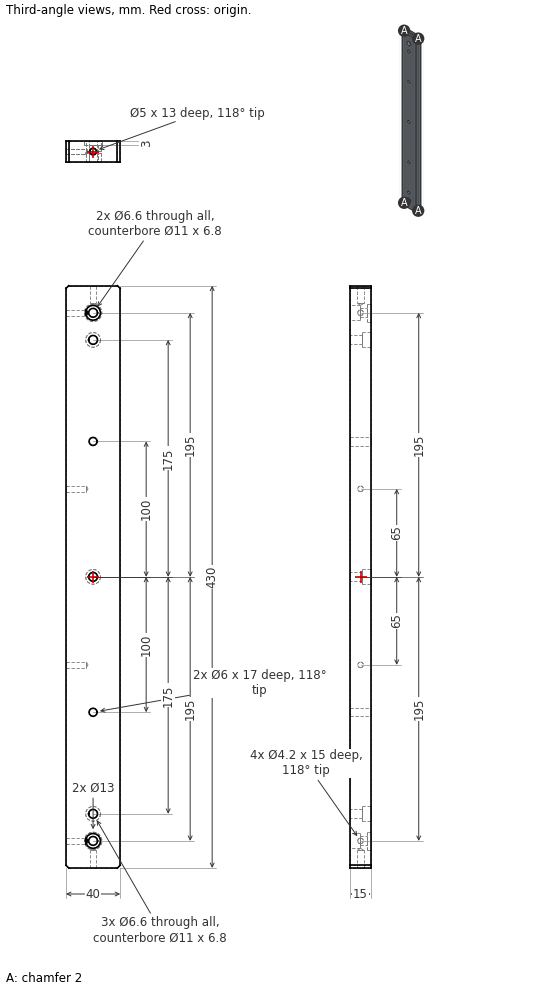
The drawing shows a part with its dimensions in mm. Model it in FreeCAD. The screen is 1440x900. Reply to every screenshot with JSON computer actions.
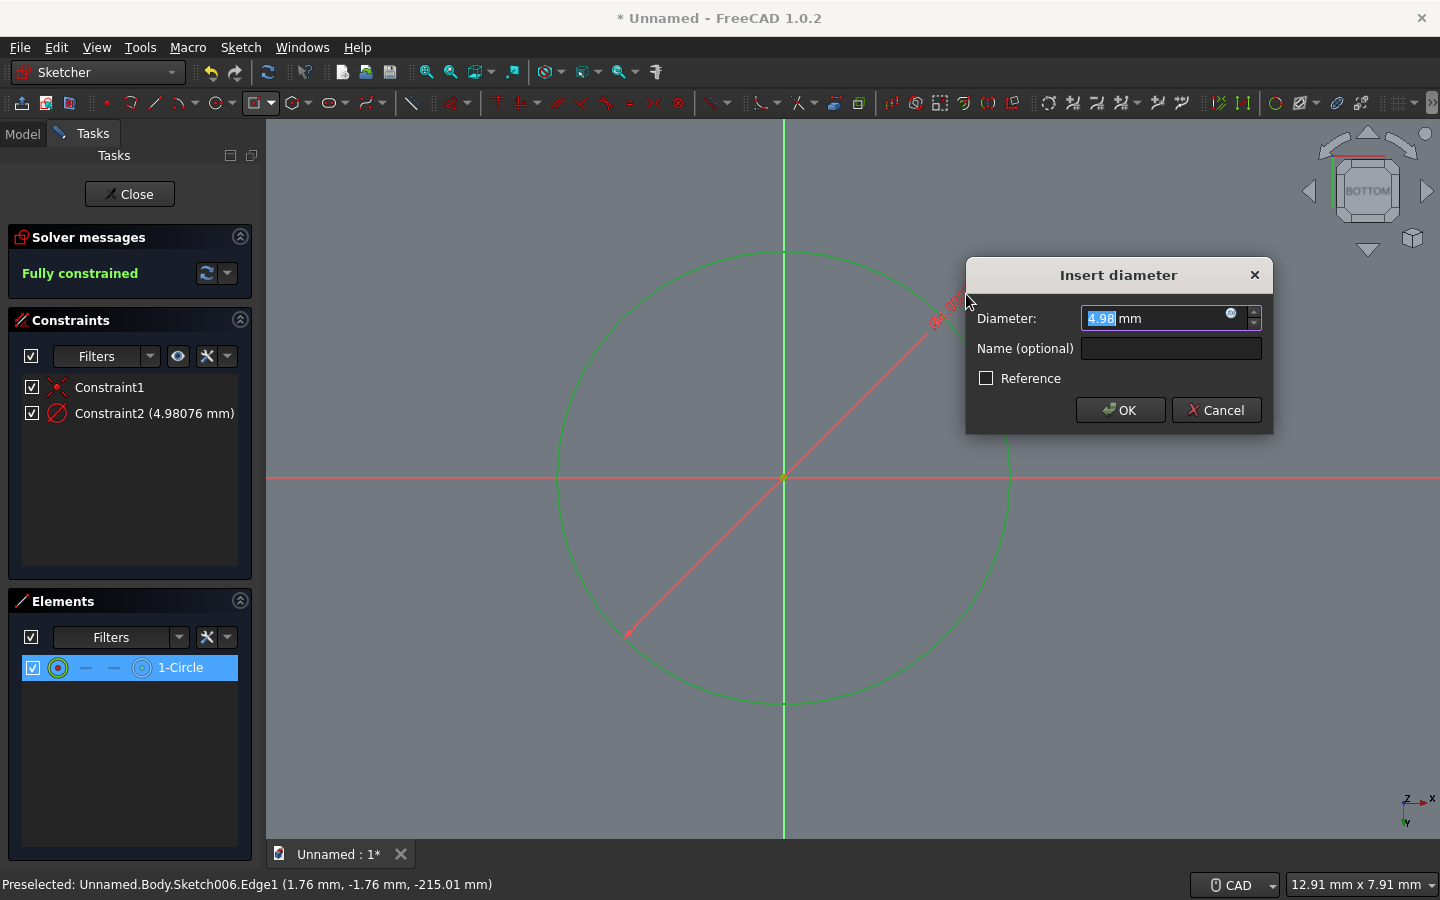
{"action": "type", "text": "5"}
{"action": "key", "text": "Return"}
{"action": "key", "text": "Escape"}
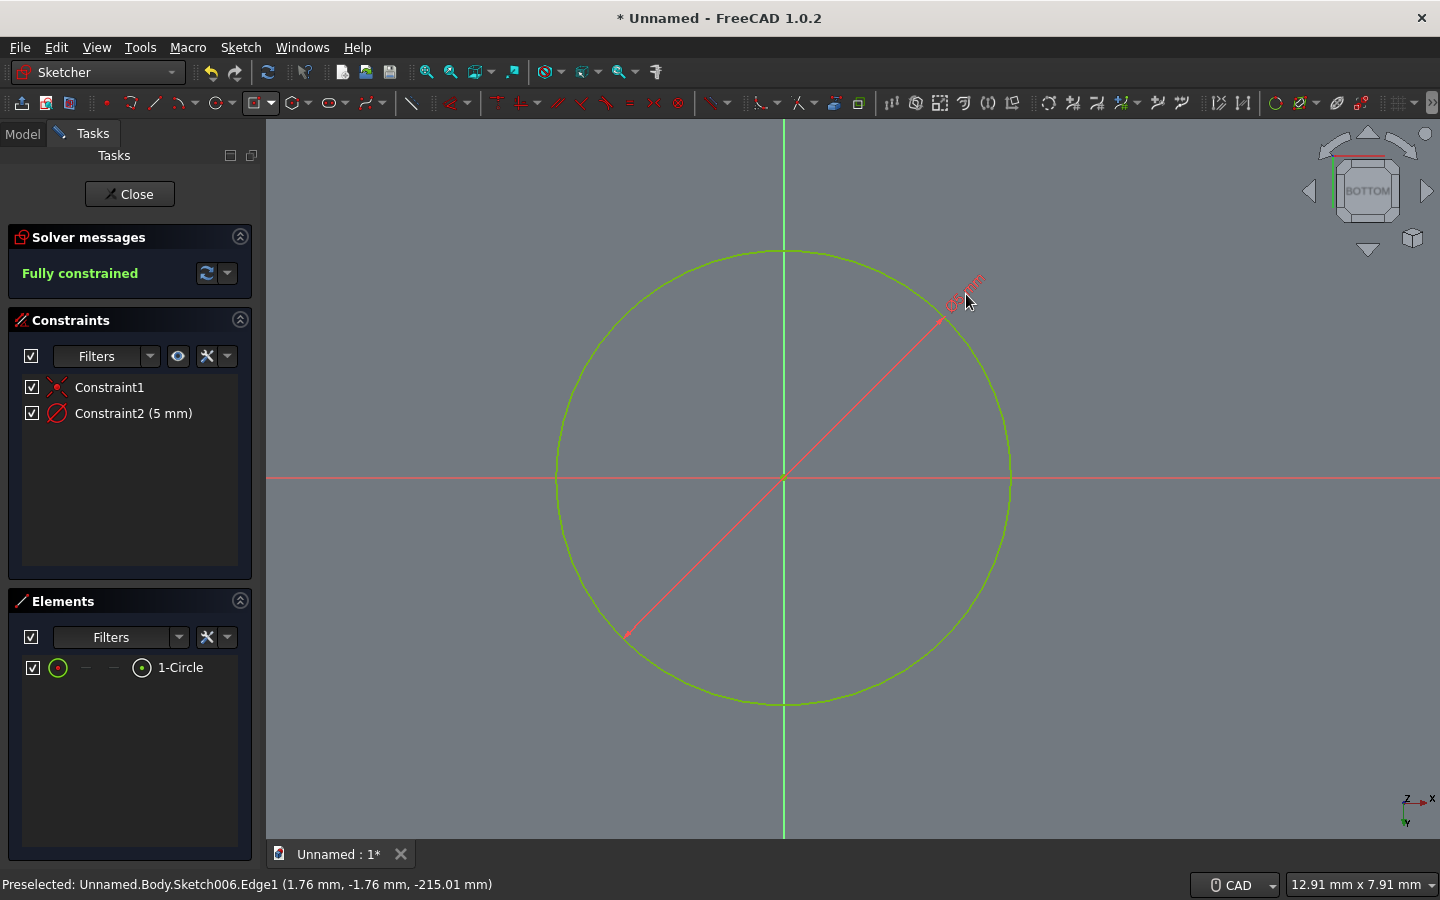
{"action": "left_click", "coordinate": [130, 194]}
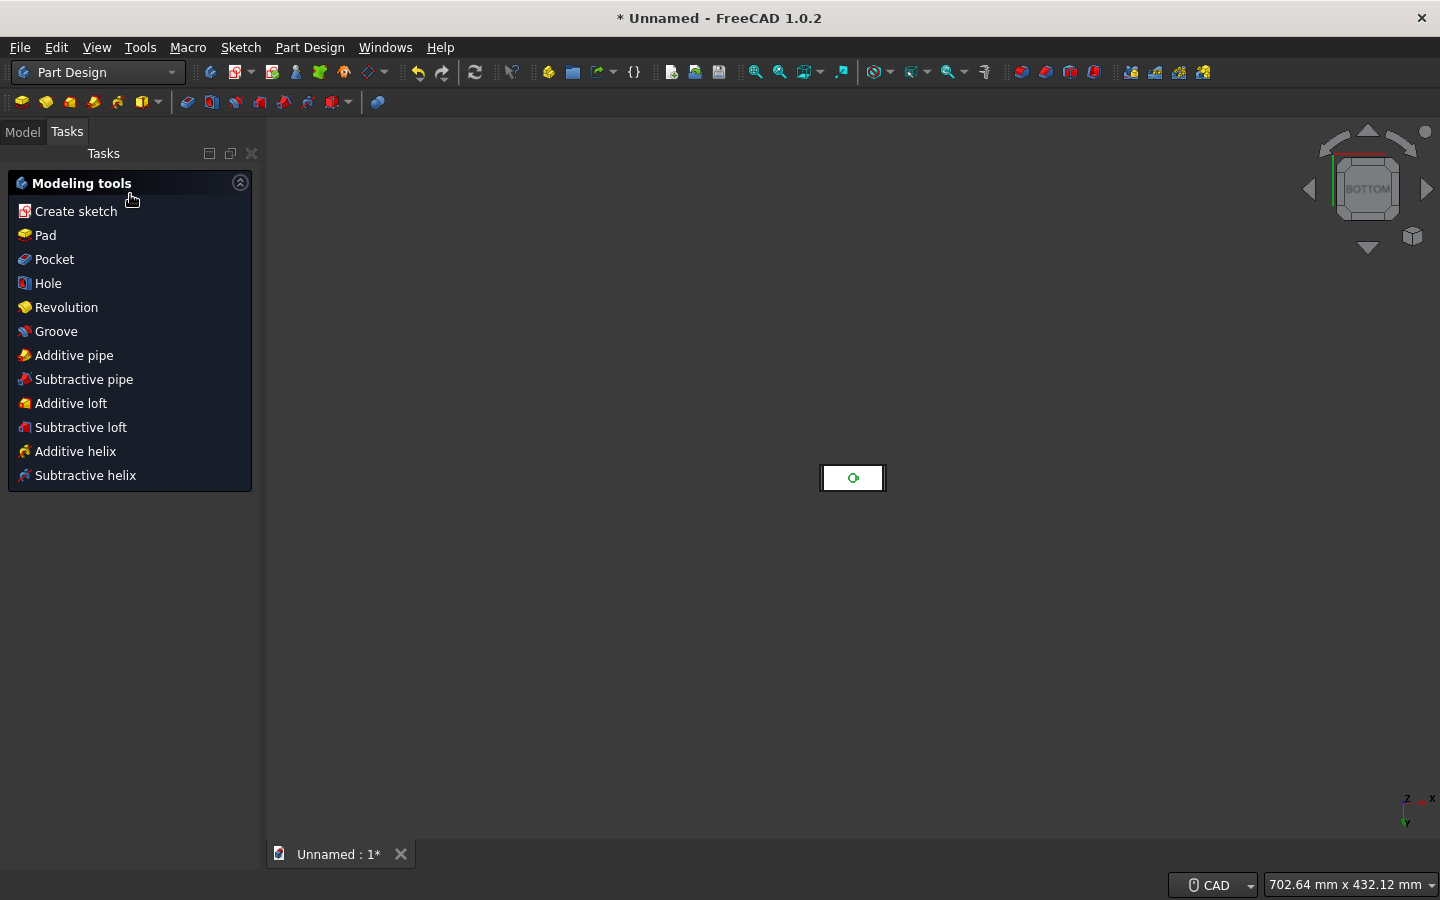
{"action": "left_click", "coordinate": [212, 102]}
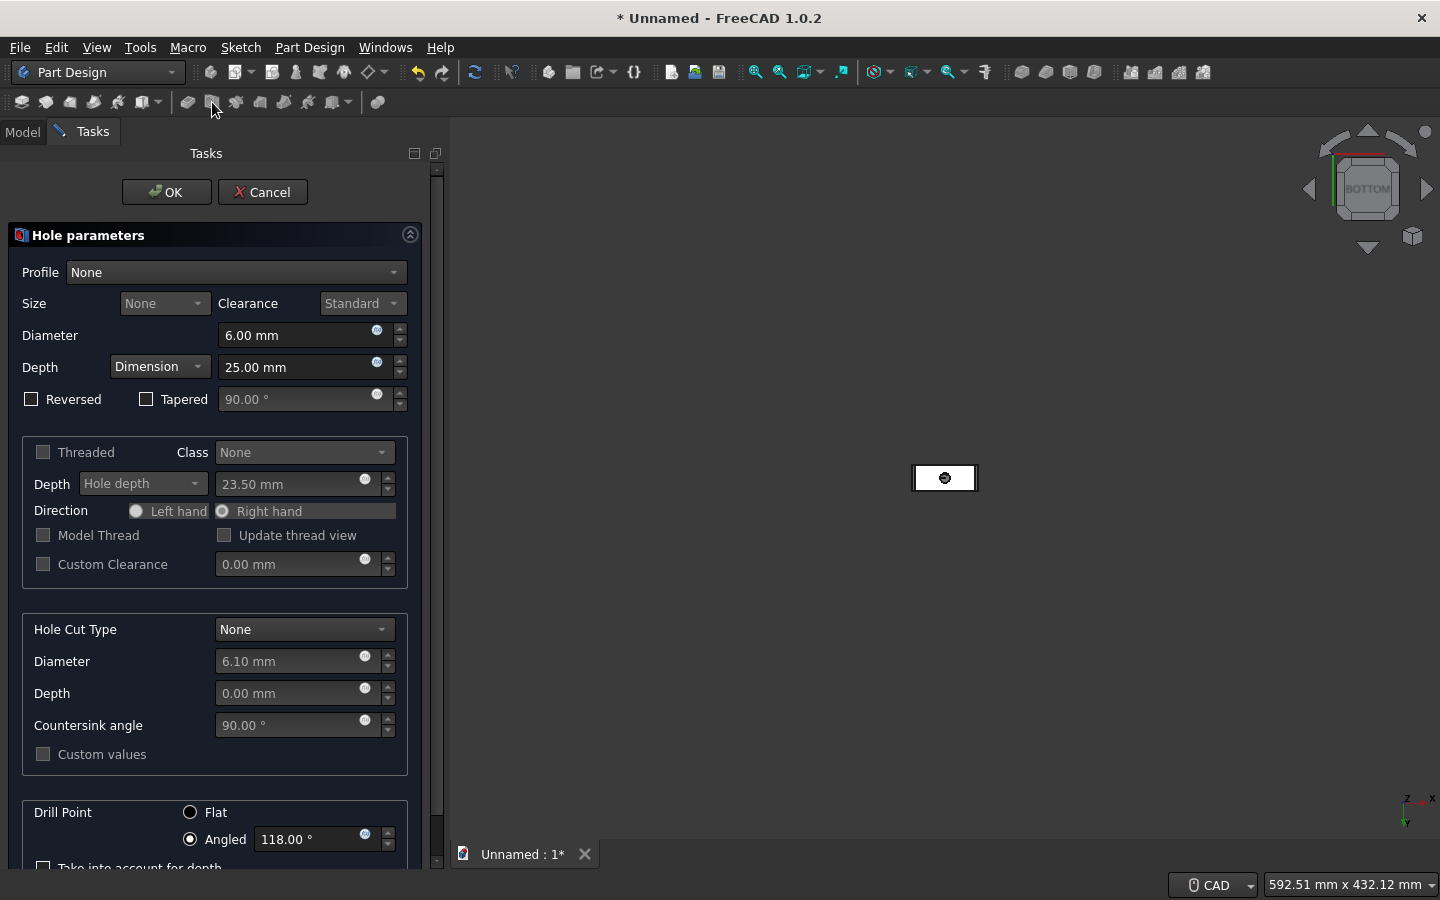
{"action": "triple_click", "coordinate": [305, 335]}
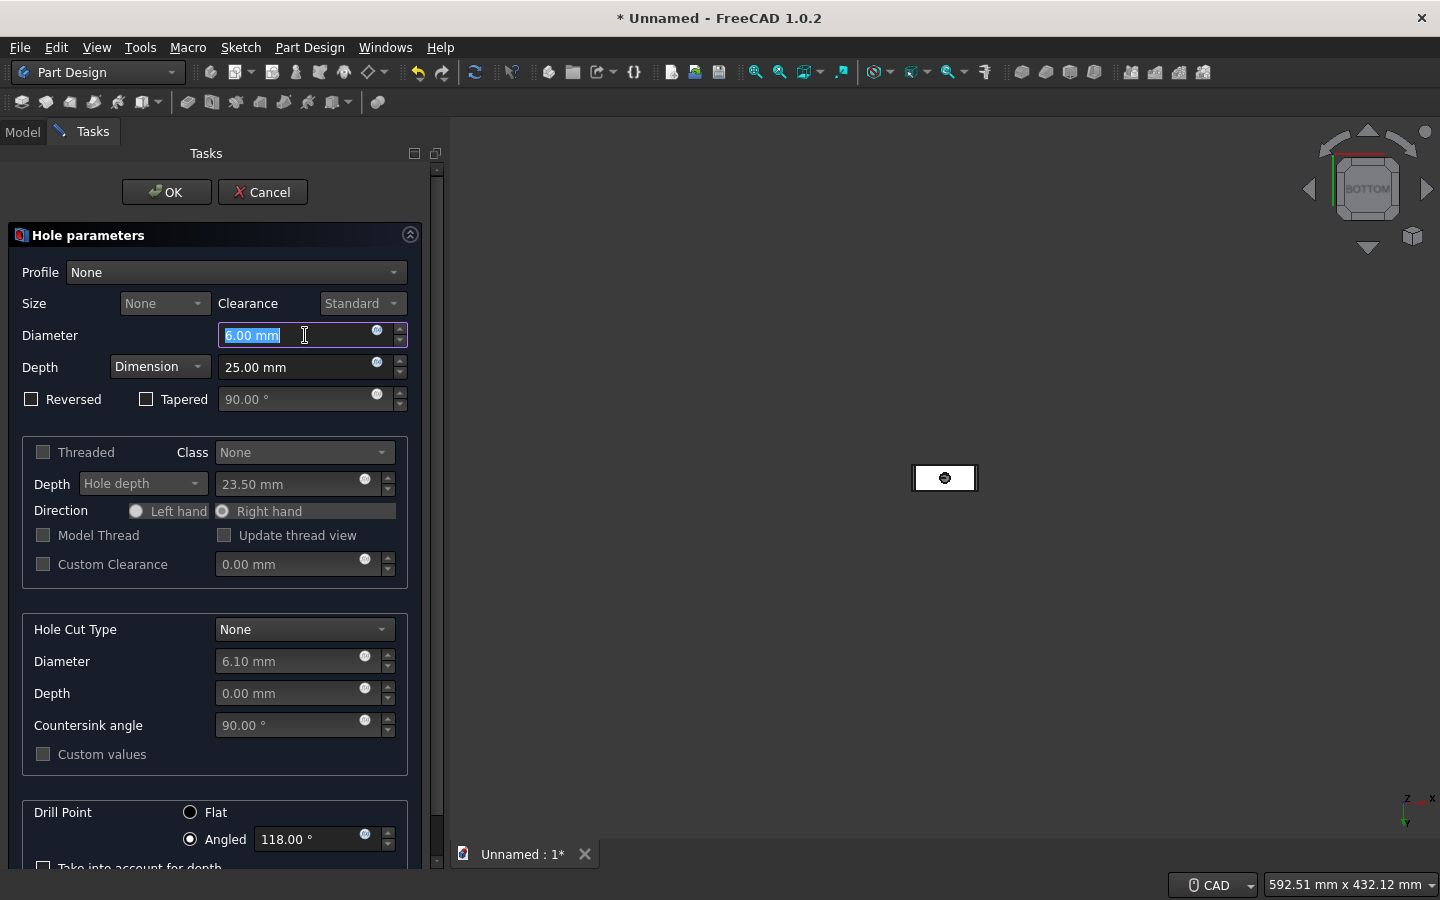
{"action": "type", "text": "5"}
{"action": "key", "text": "Tab"}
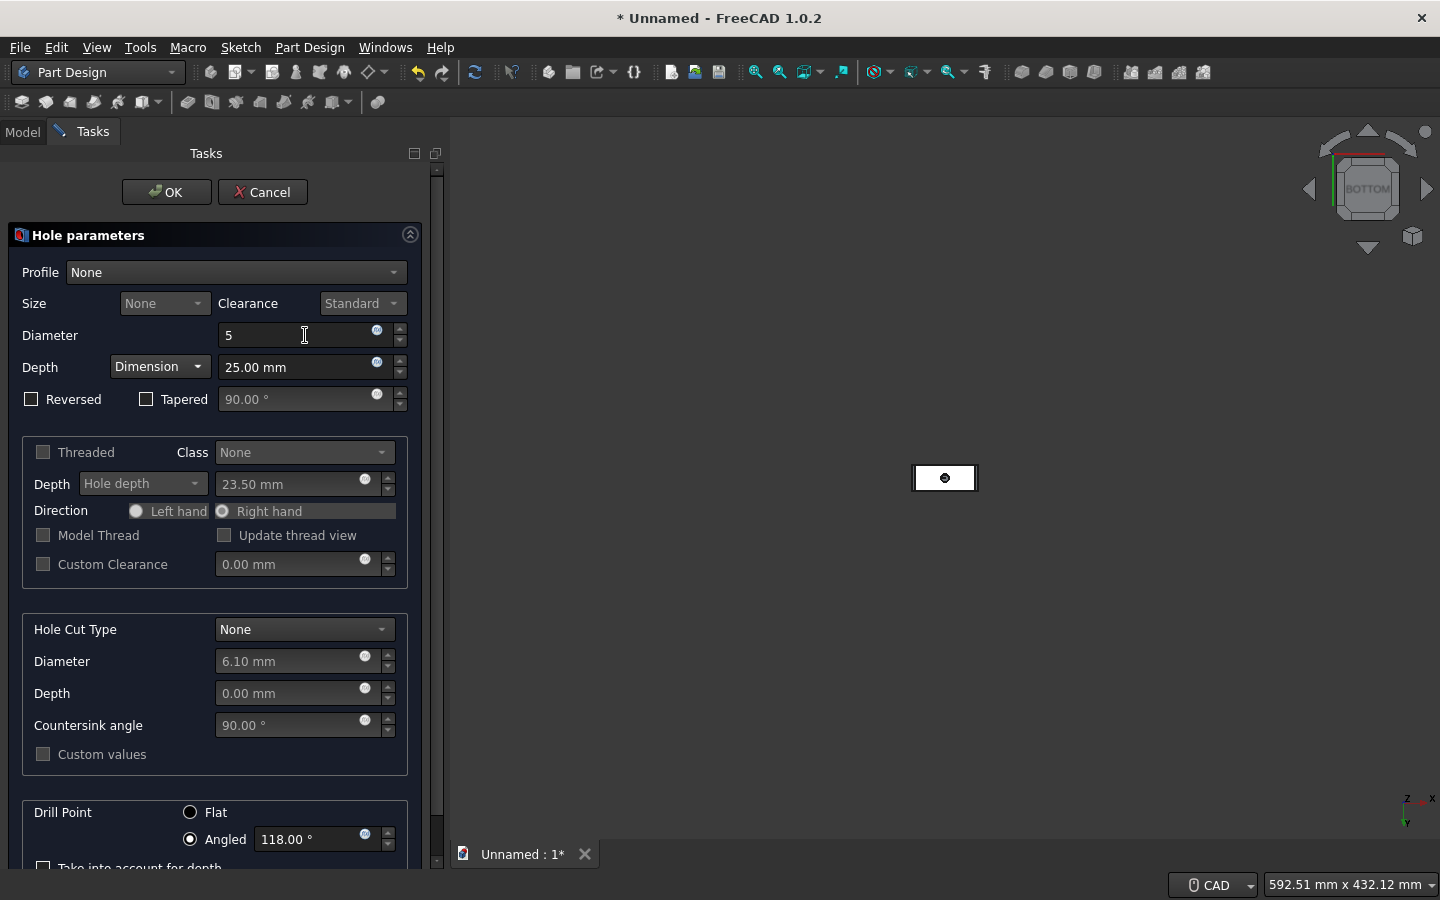
{"action": "triple_click", "coordinate": [305, 367]}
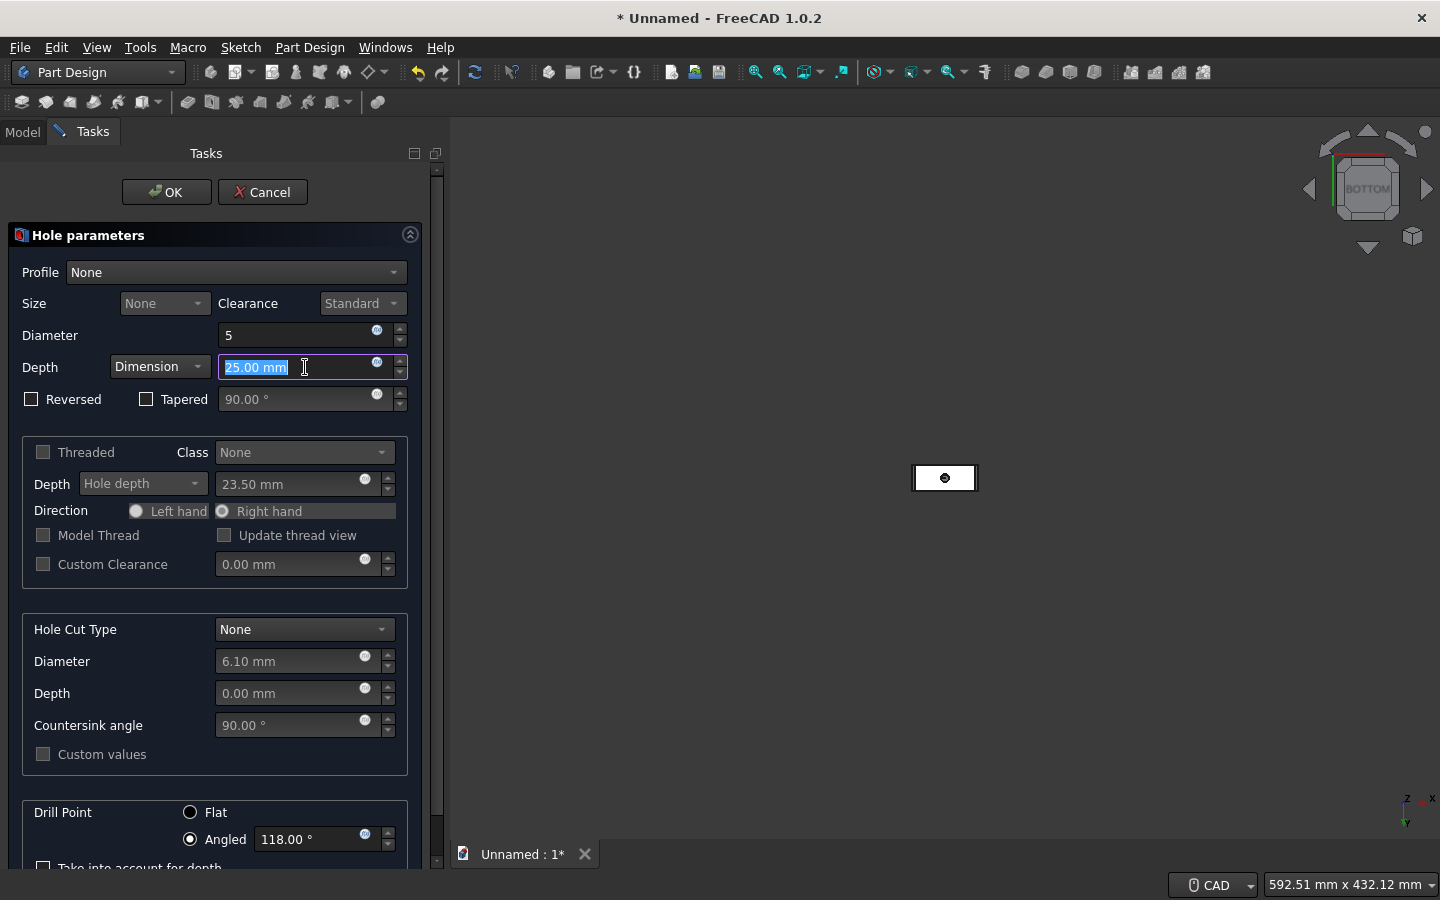
{"action": "type", "text": "13"}
{"action": "key", "text": "Tab"}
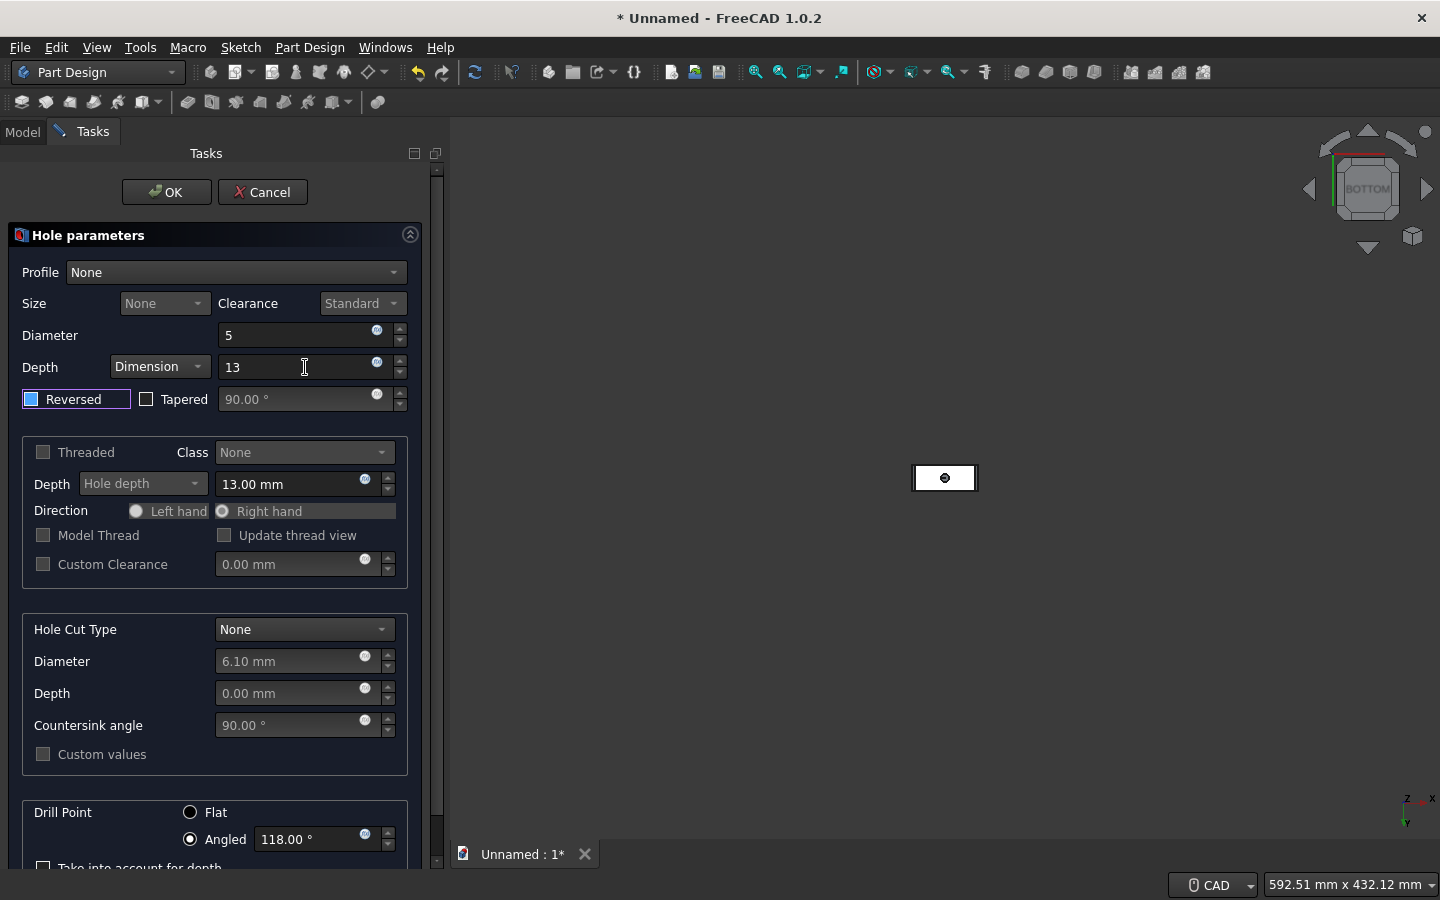
{"action": "left_click", "coordinate": [167, 192]}